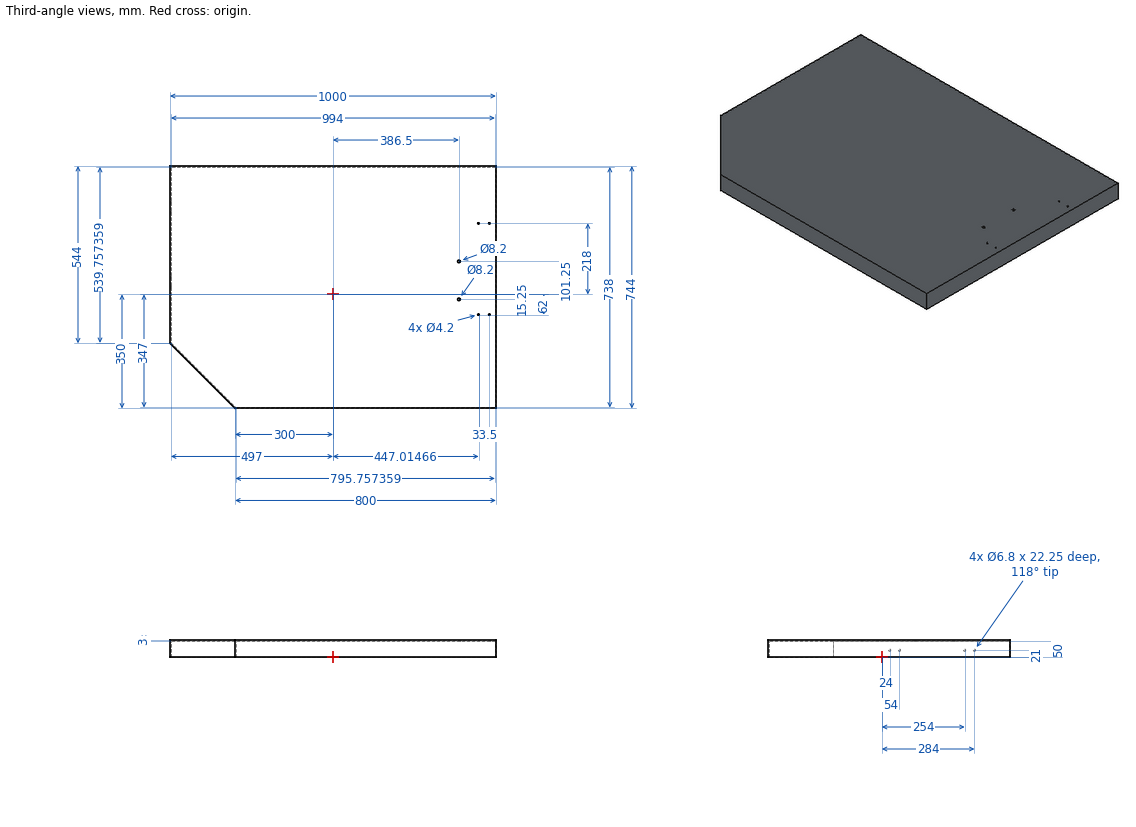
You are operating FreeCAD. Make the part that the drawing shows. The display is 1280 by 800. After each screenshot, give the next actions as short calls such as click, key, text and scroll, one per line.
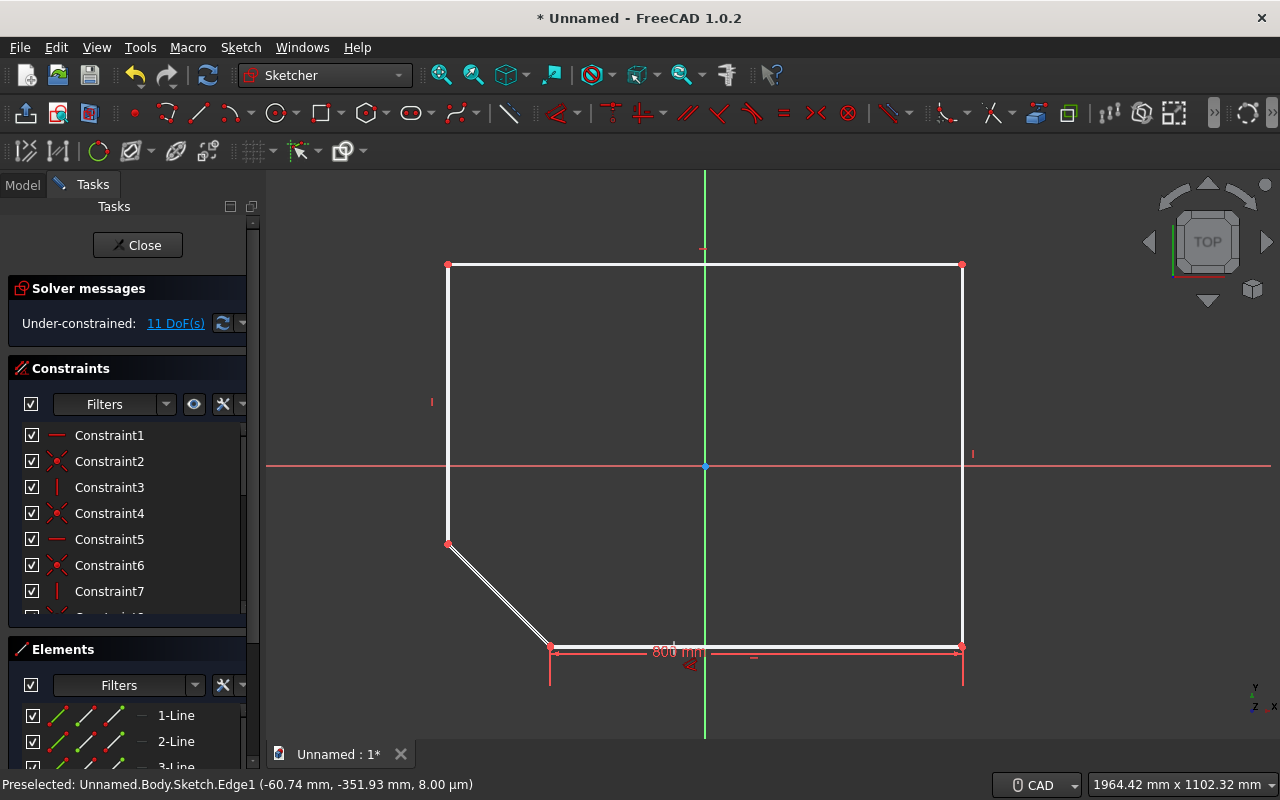
scroll(963, 533, up, 12)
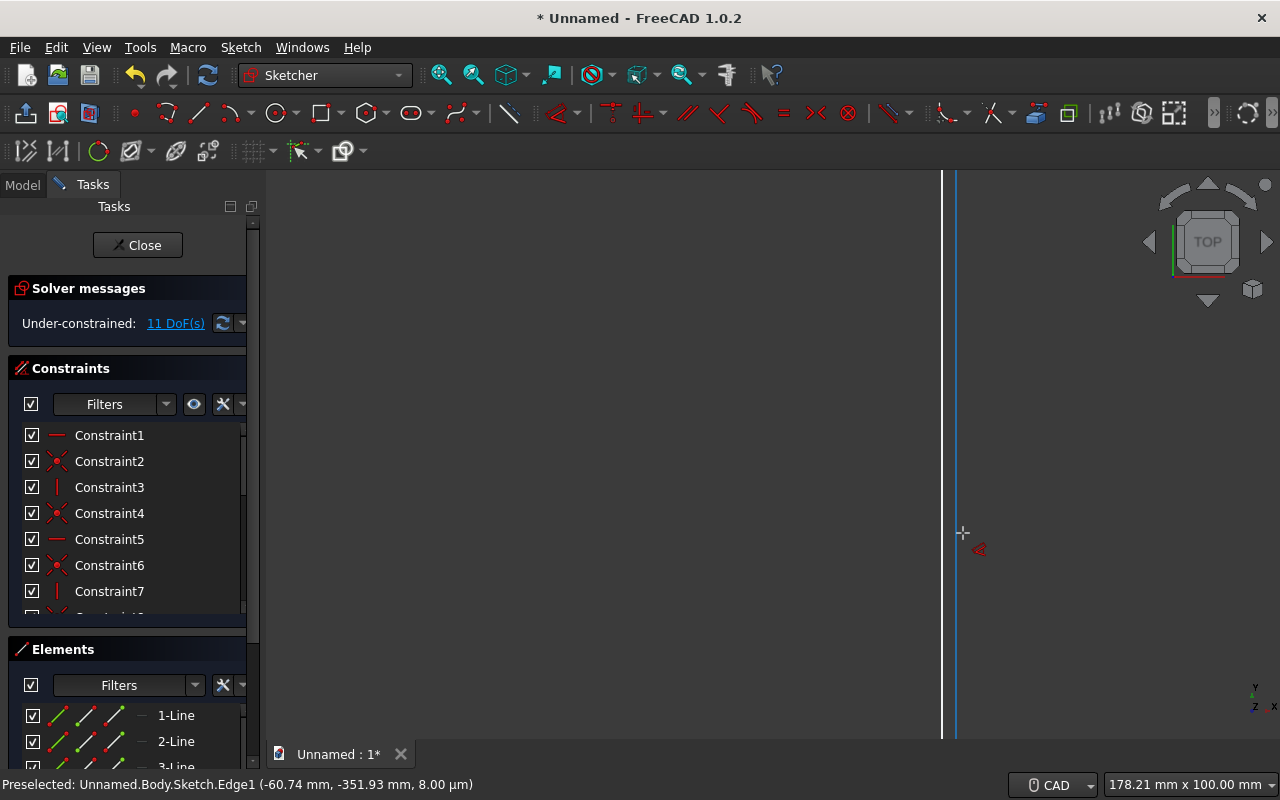
click(956, 524)
click(990, 454)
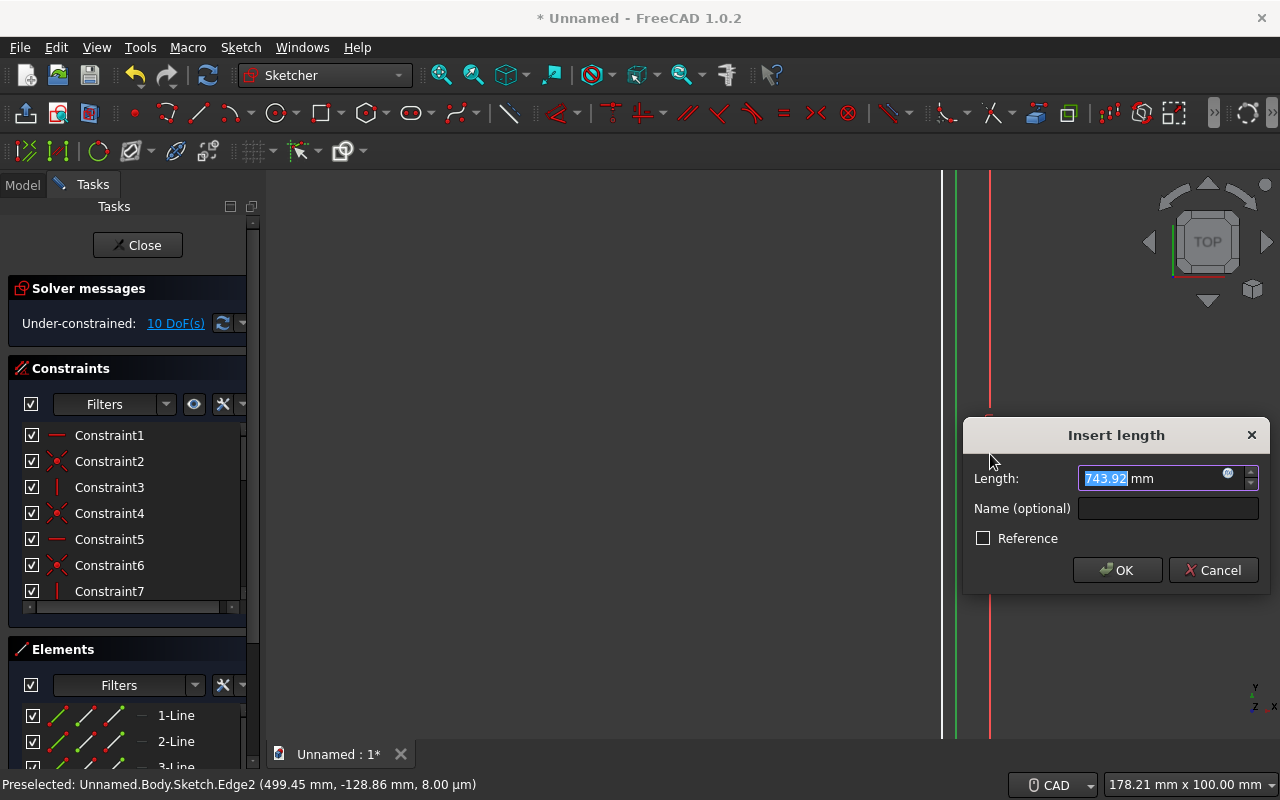
text(744)
key(Return)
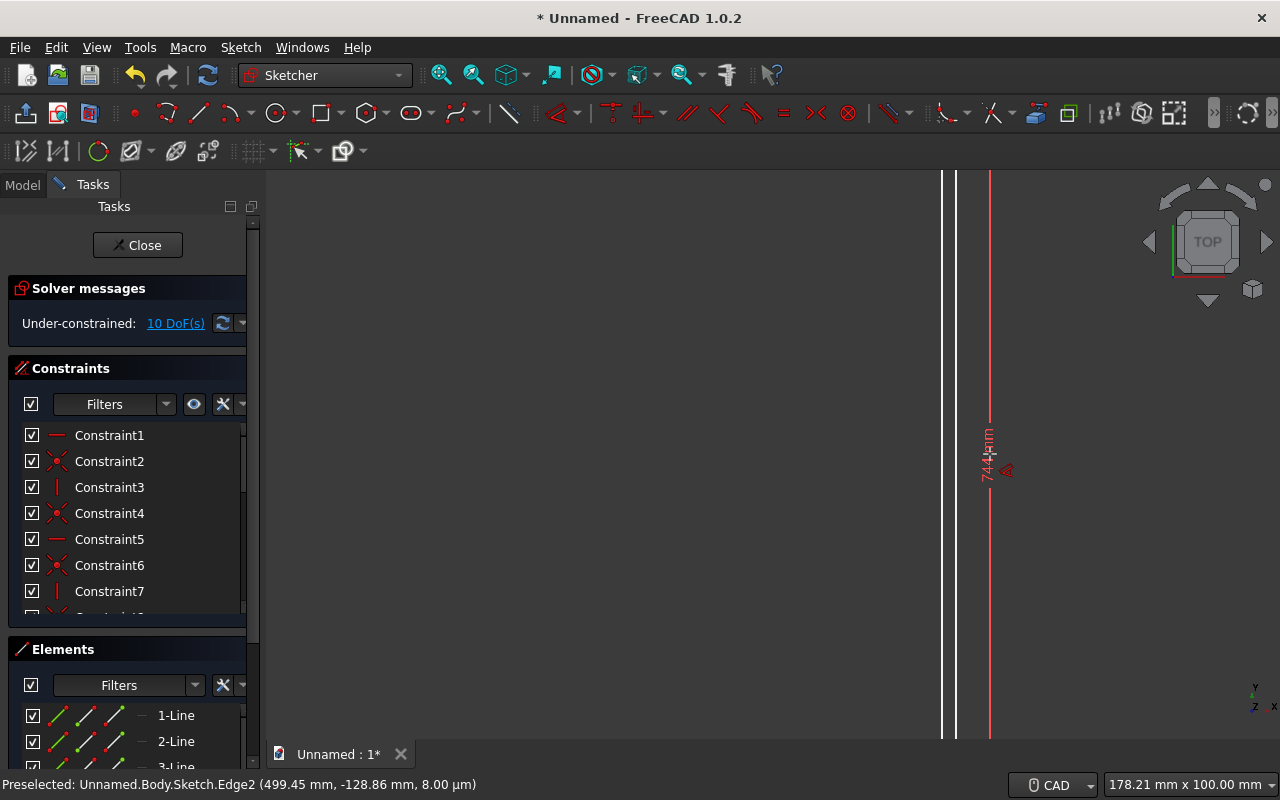
scroll(963, 533, down, 12)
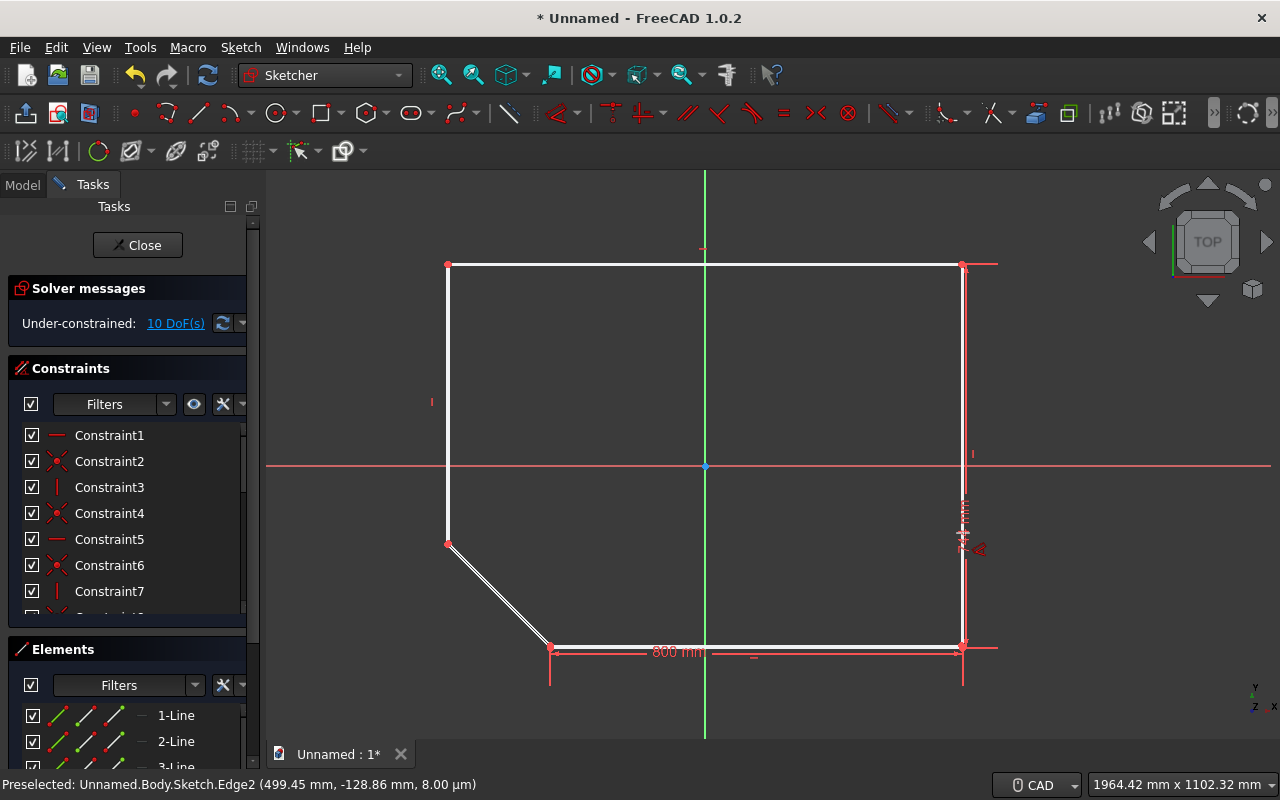
scroll(447, 348, up, 11)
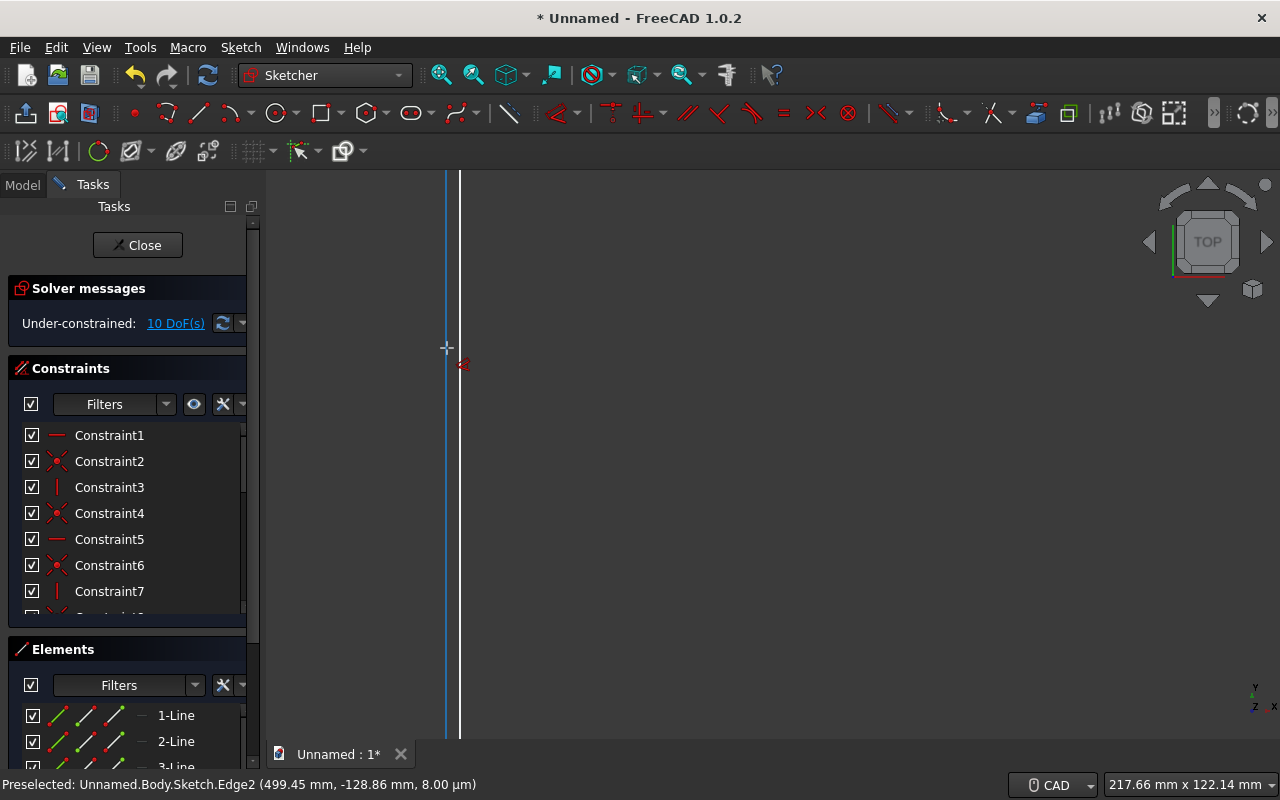
click(446, 348)
click(412, 454)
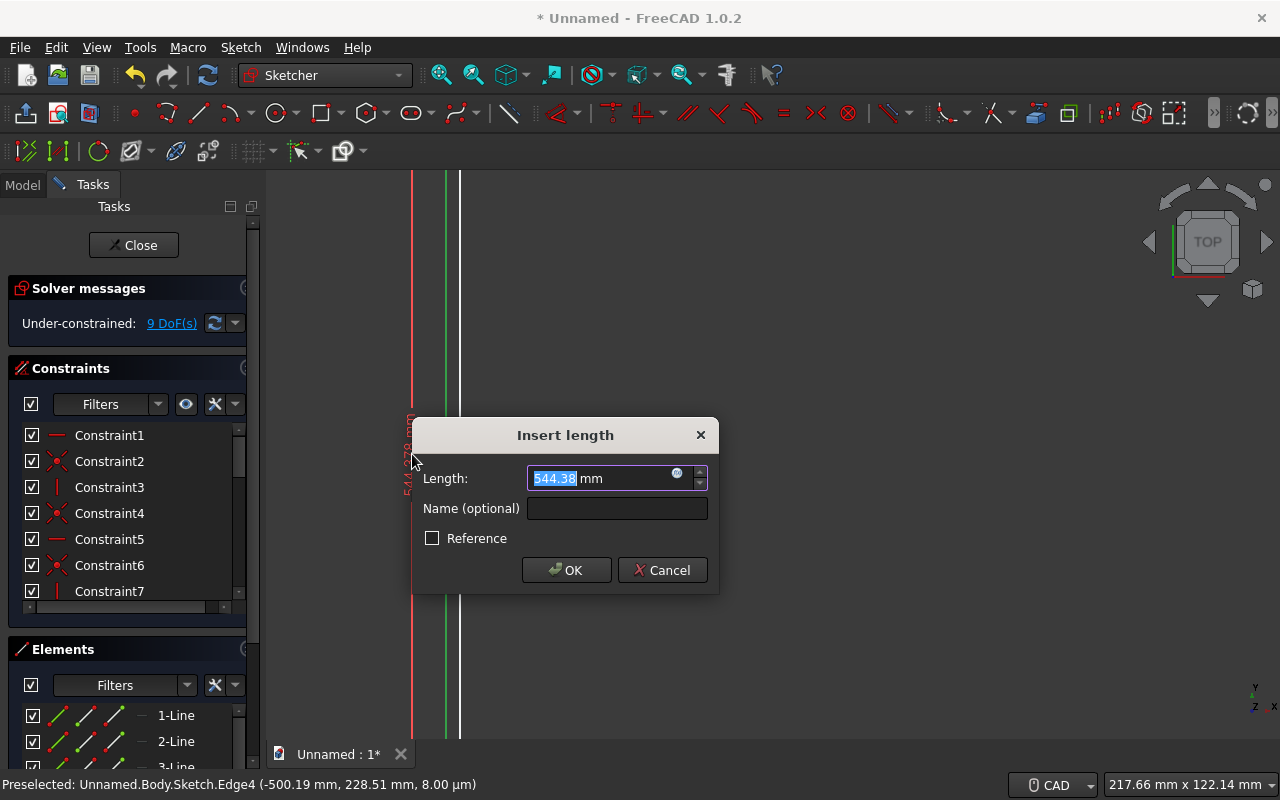
text(544)
key(Return)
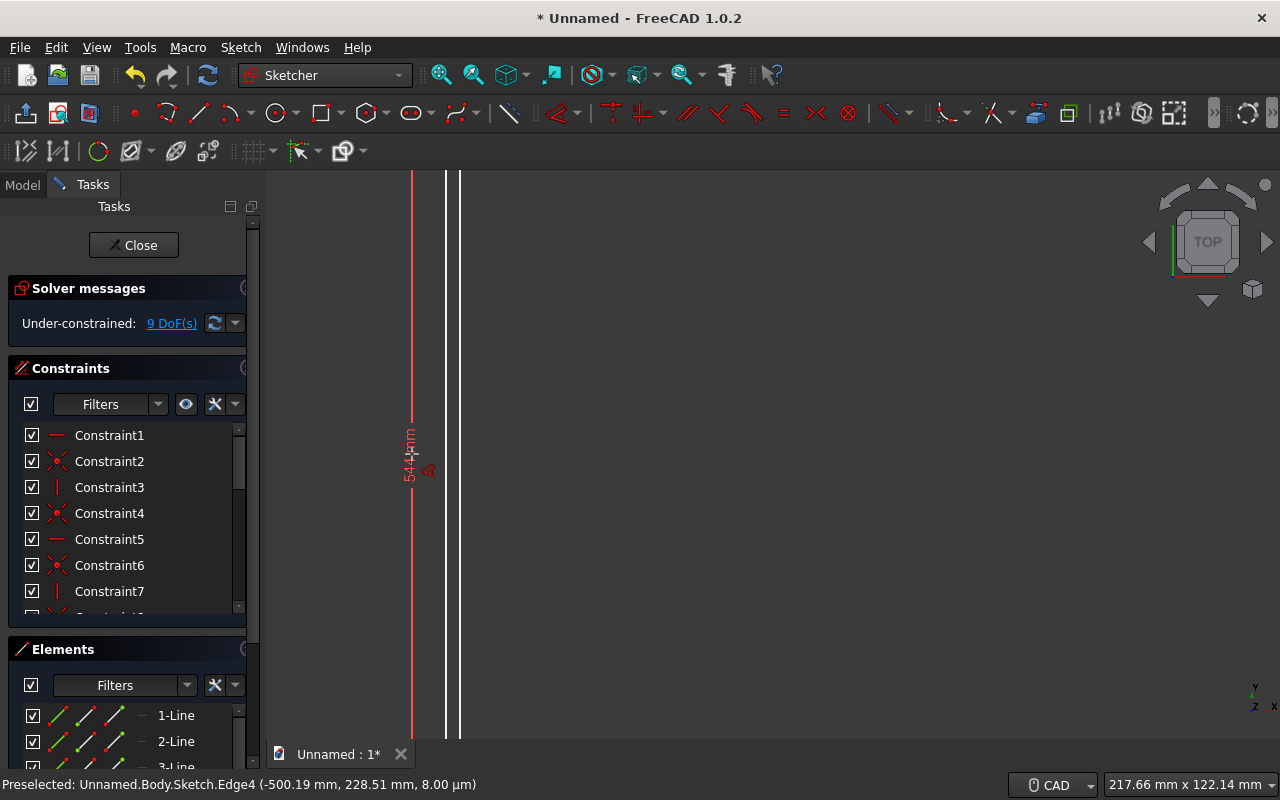
scroll(446, 348, down, 11)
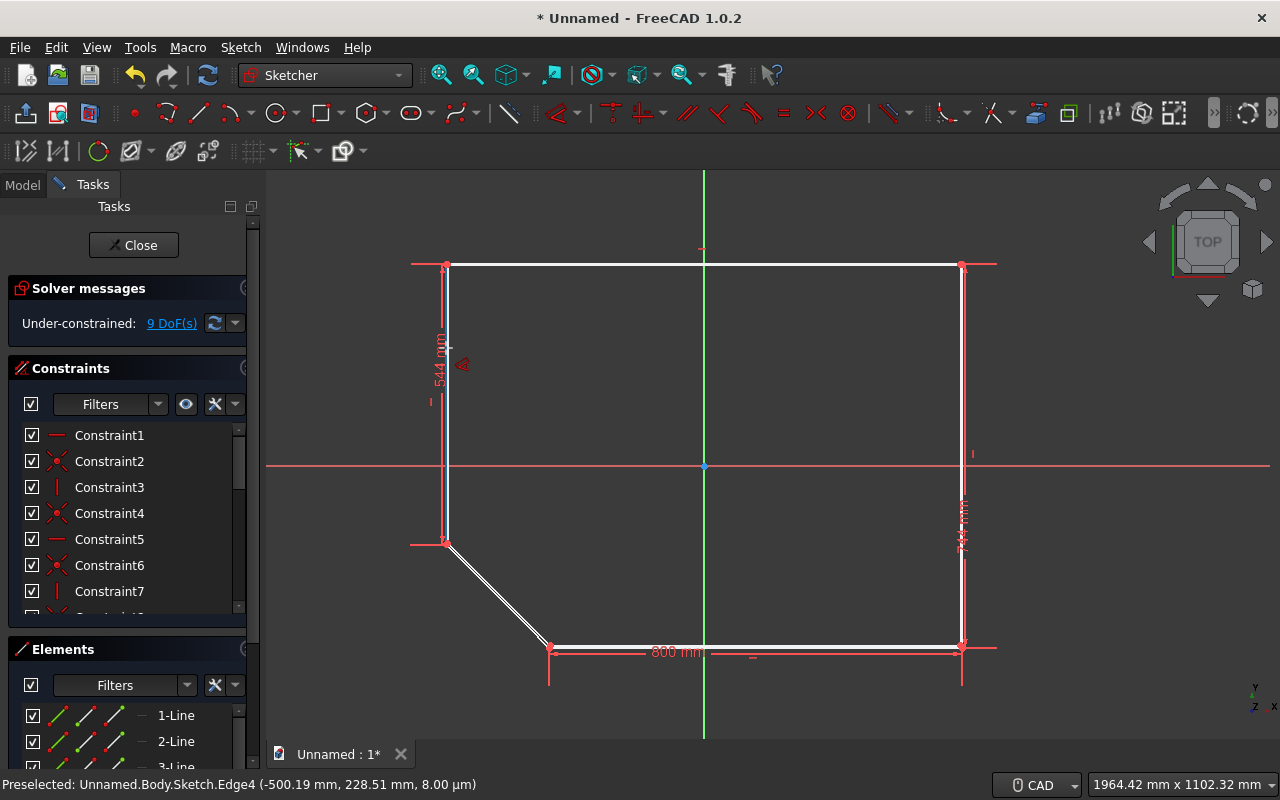
scroll(602, 265, up, 14)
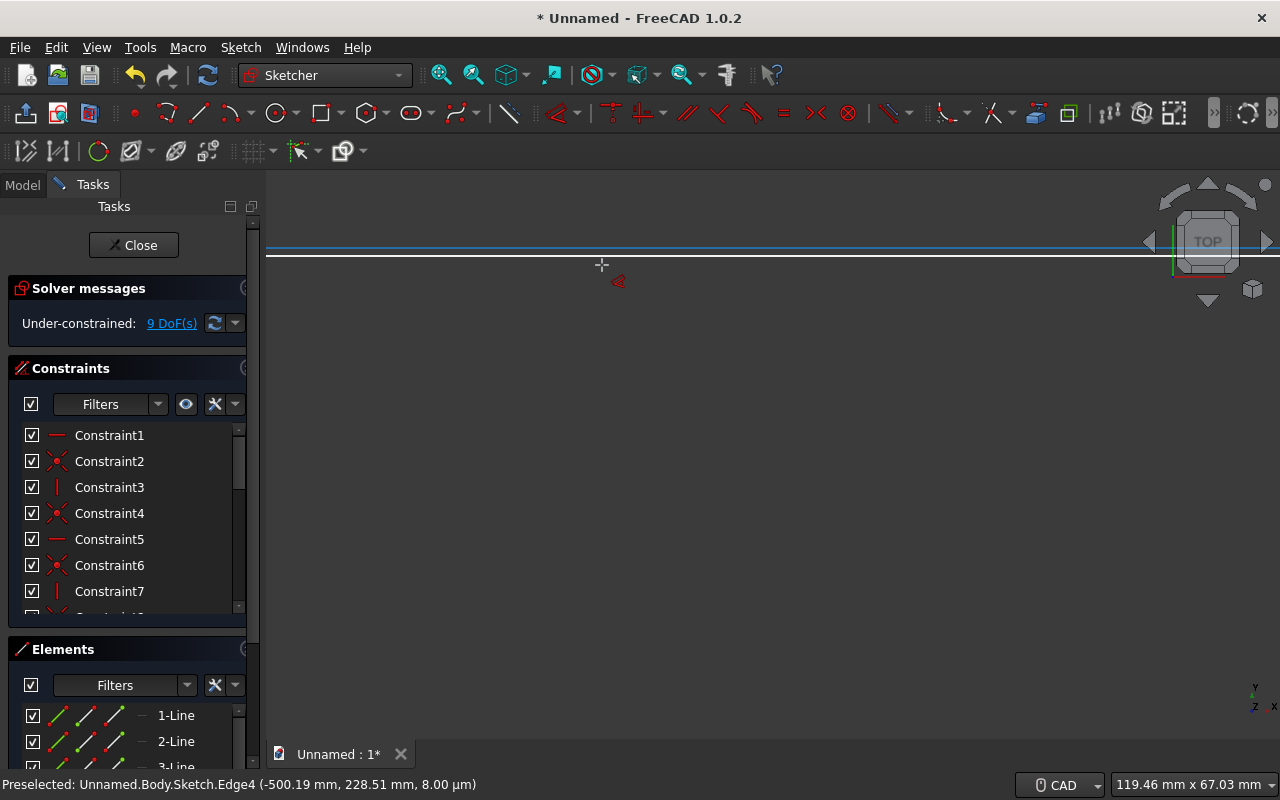
click(591, 256)
click(704, 222)